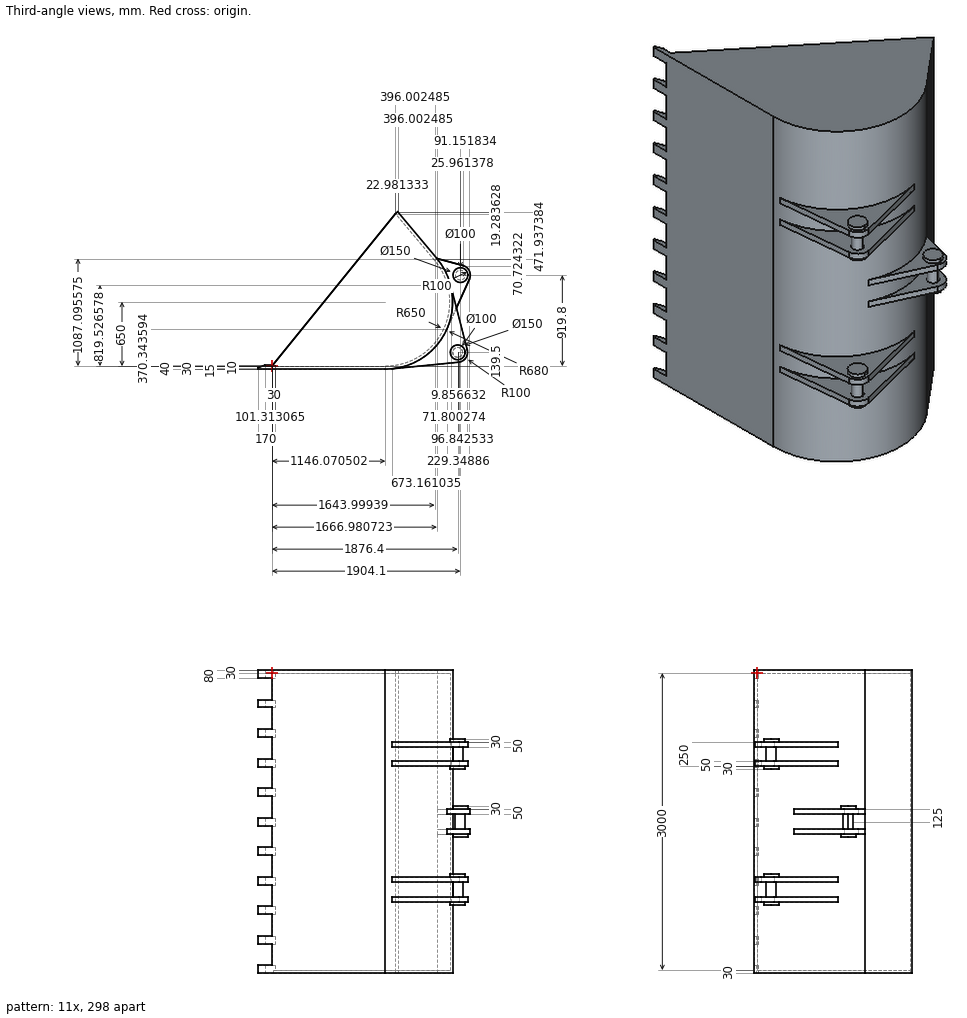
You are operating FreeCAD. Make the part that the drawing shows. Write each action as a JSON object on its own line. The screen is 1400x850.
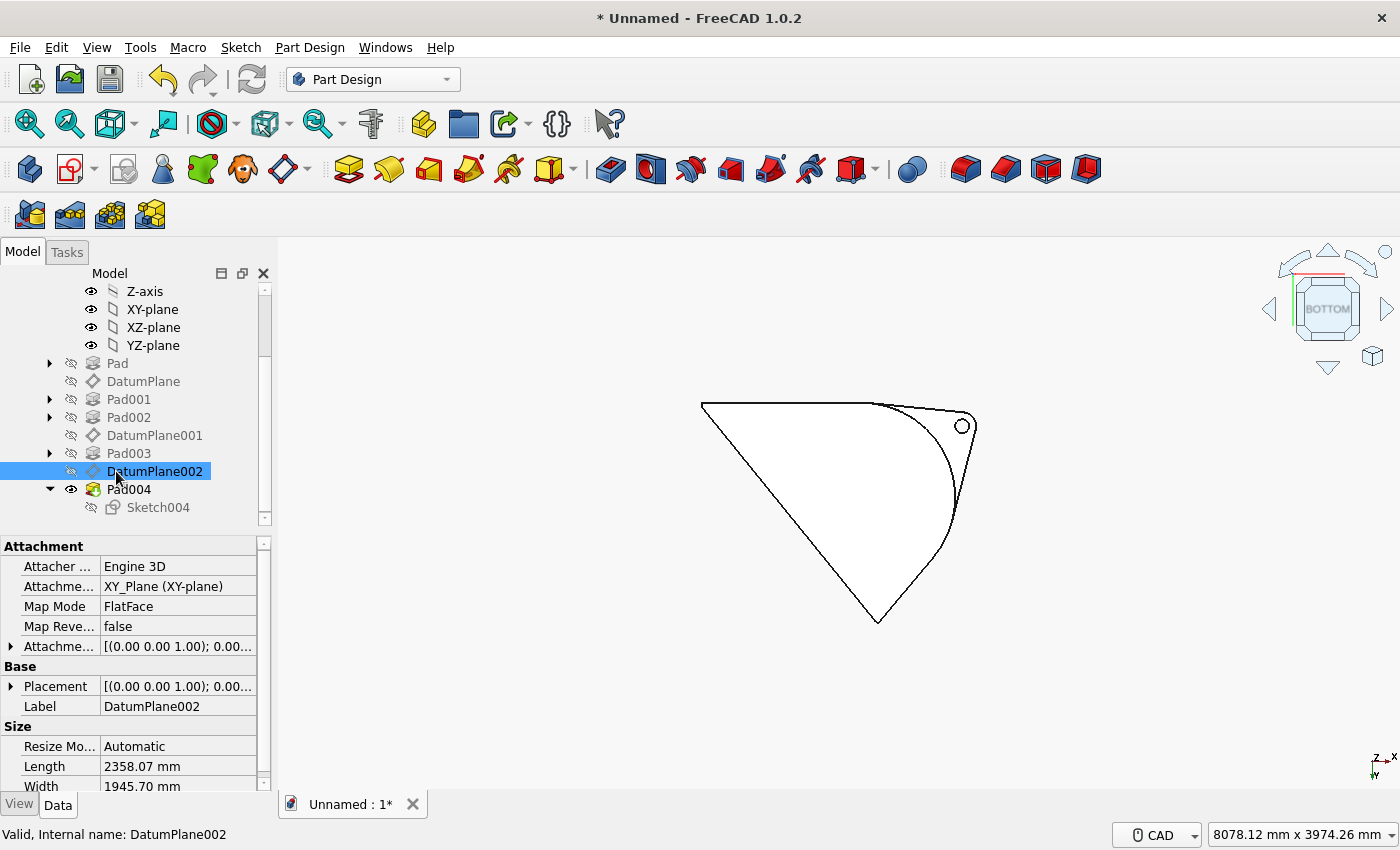
{"action": "left_click", "coordinate": [30, 124]}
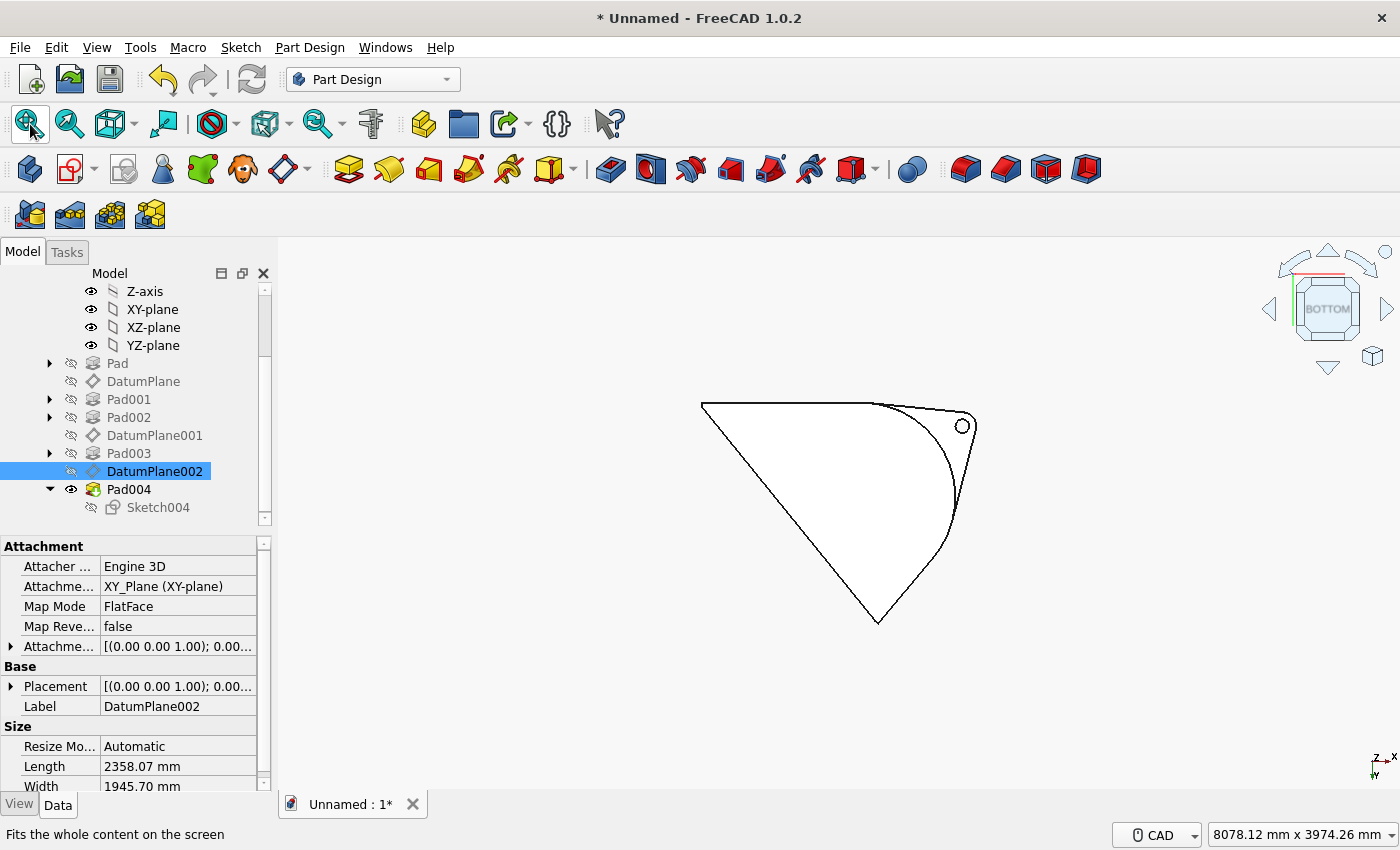
{"action": "scroll", "coordinate": [160, 395], "scroll_direction": "down", "scroll_amount": 3}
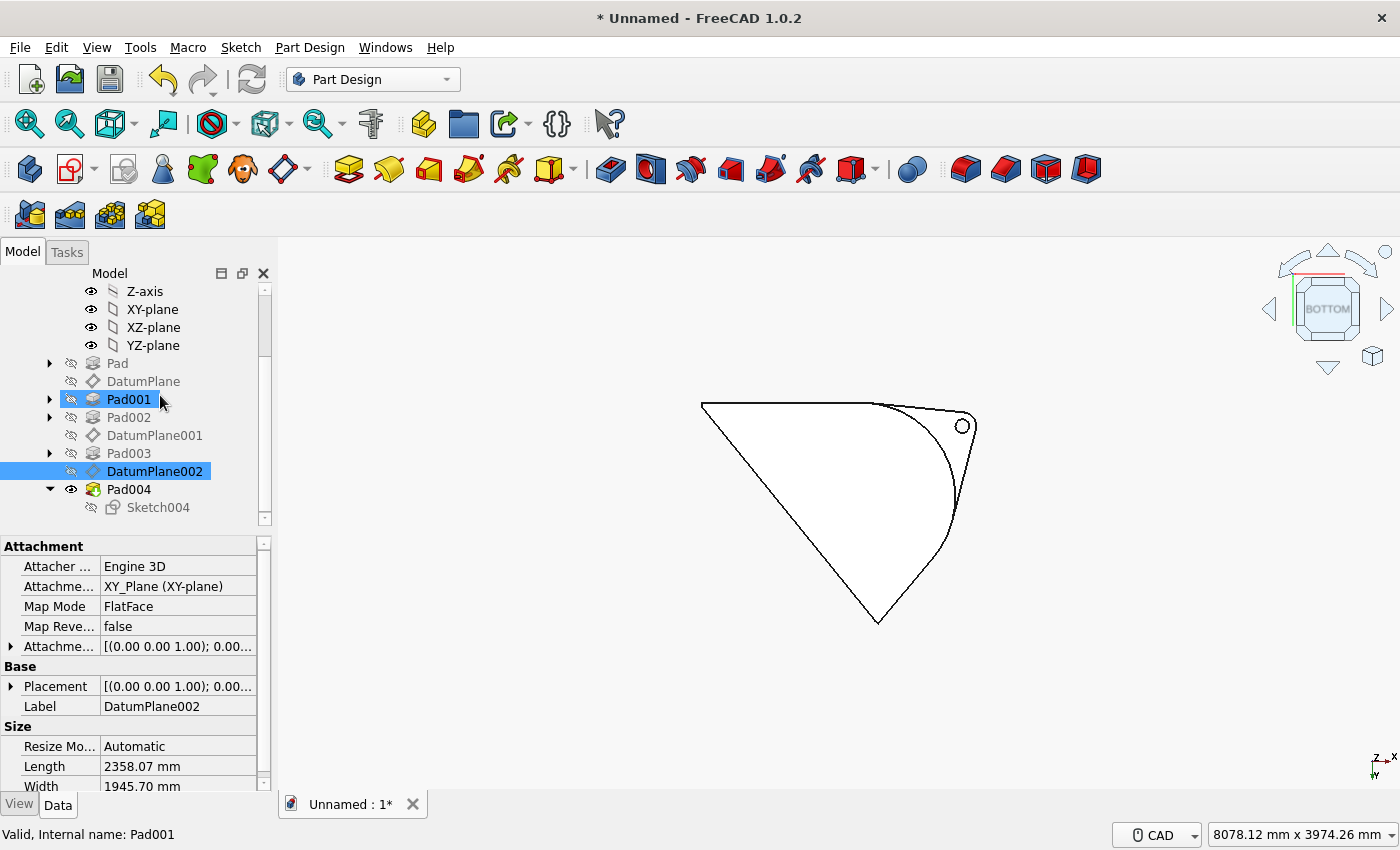
{"action": "scroll", "coordinate": [160, 395], "scroll_direction": "up", "scroll_amount": 15}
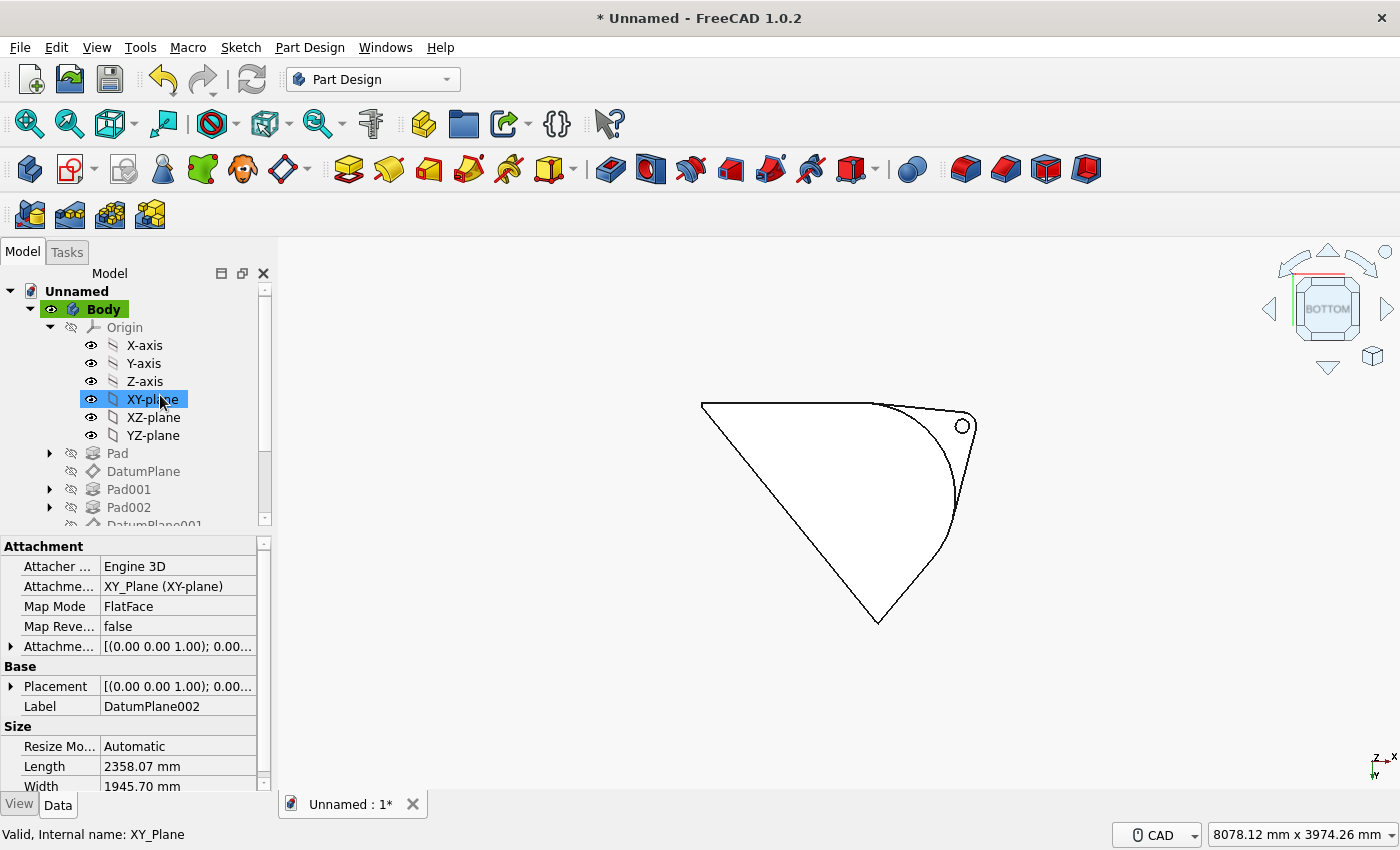
{"action": "left_click", "coordinate": [136, 399]}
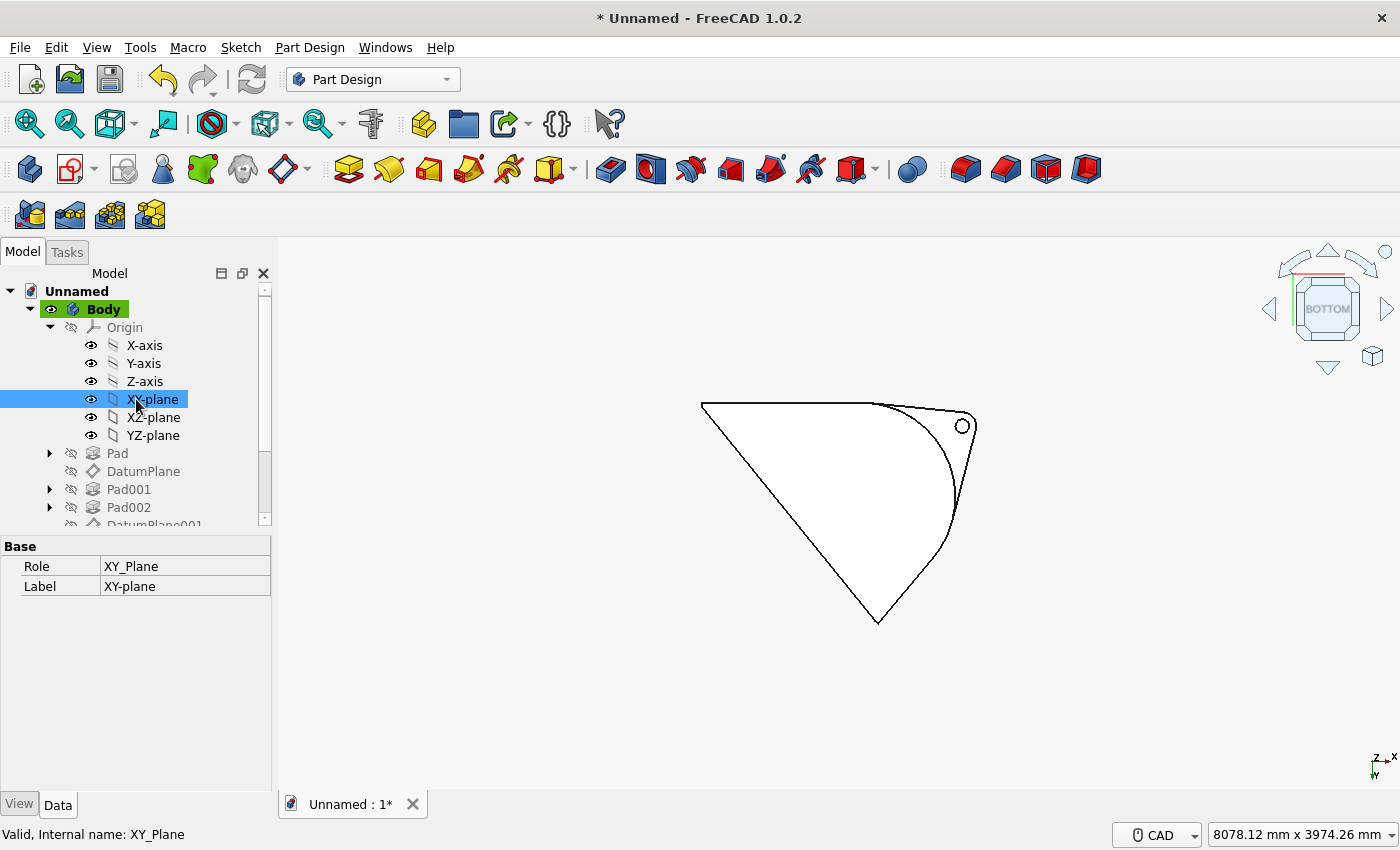
{"action": "left_click", "coordinate": [284, 170]}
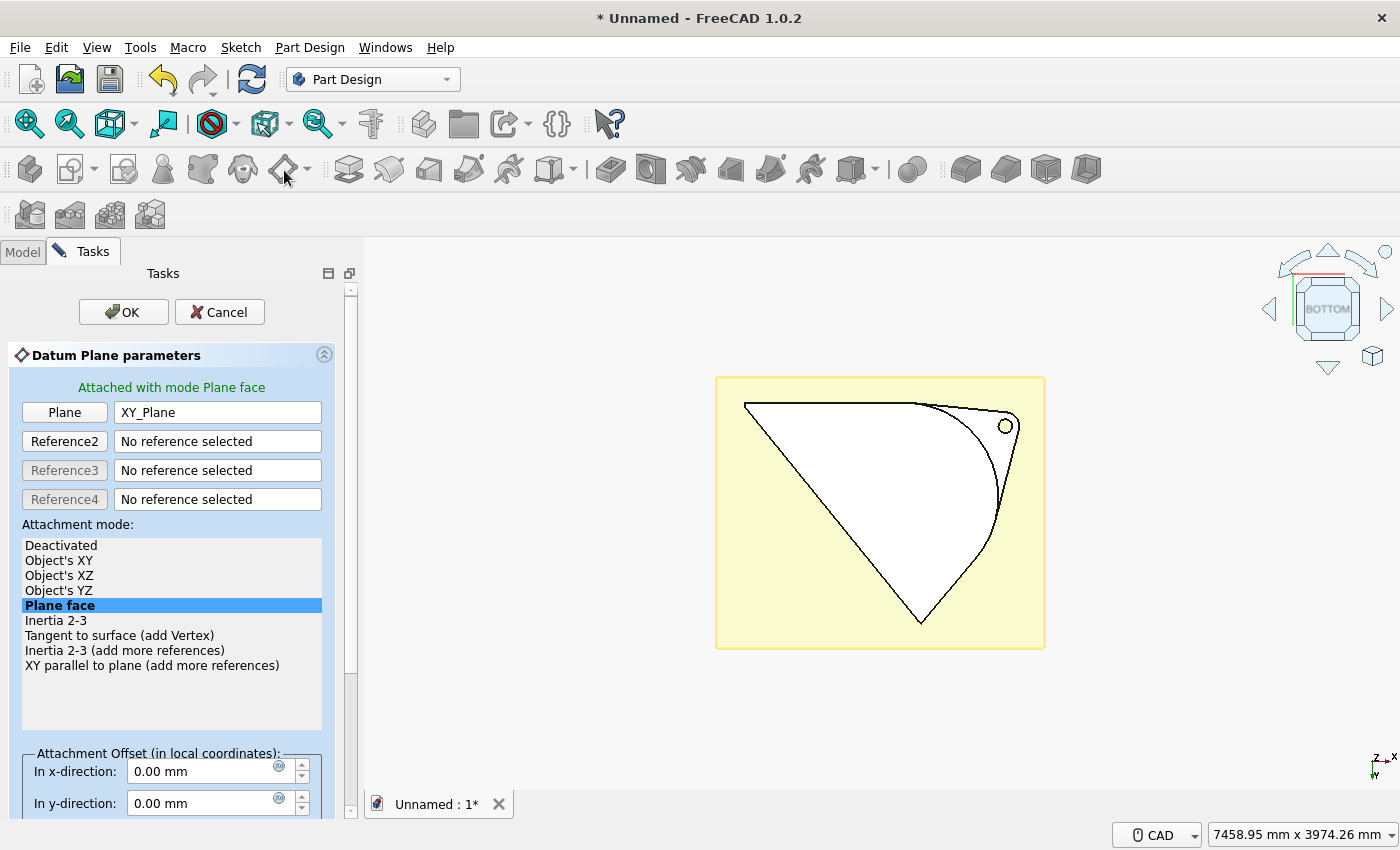
{"action": "scroll", "coordinate": [351, 550], "scroll_direction": "down", "scroll_amount": 2}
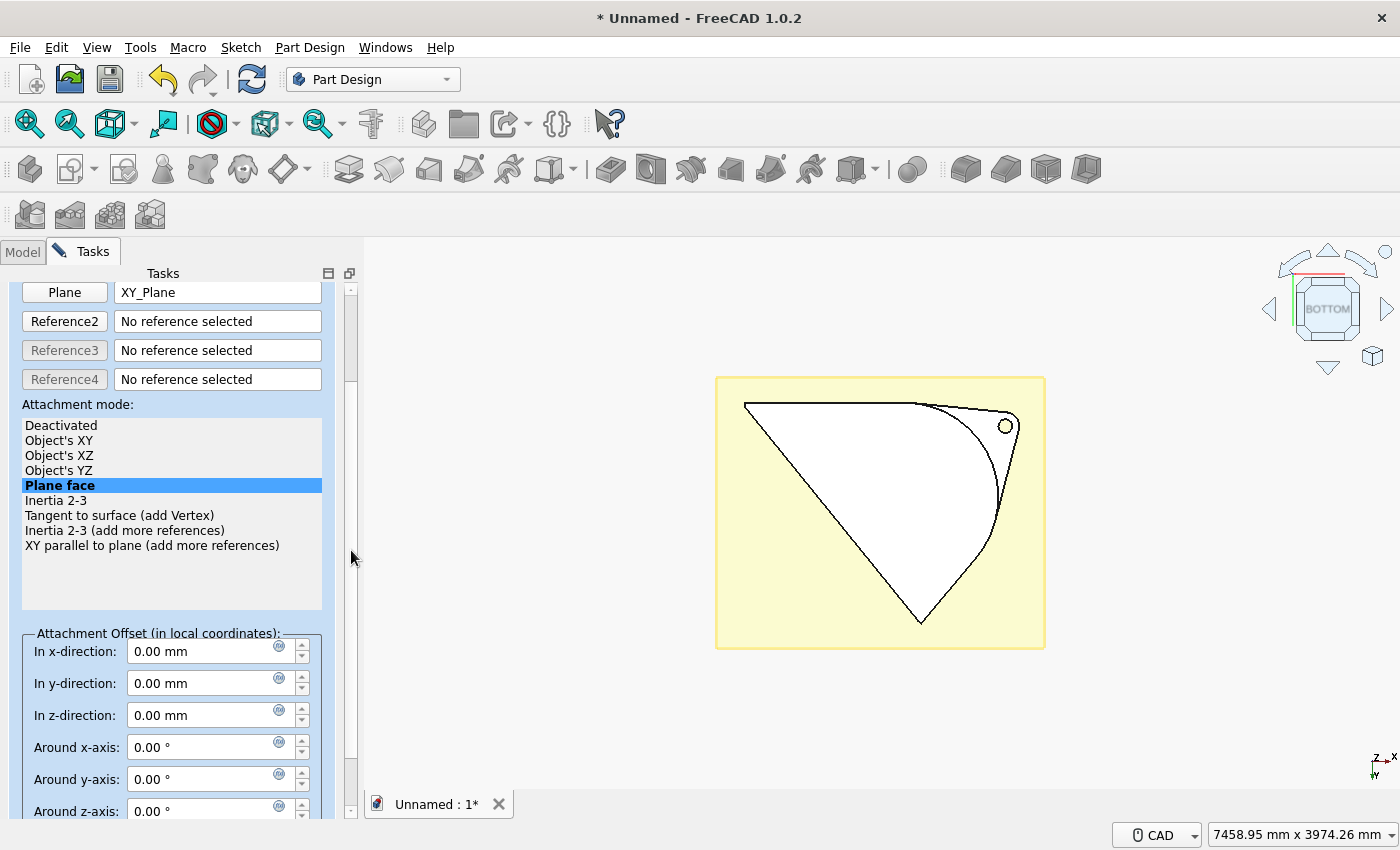
{"action": "triple_click", "coordinate": [210, 715]}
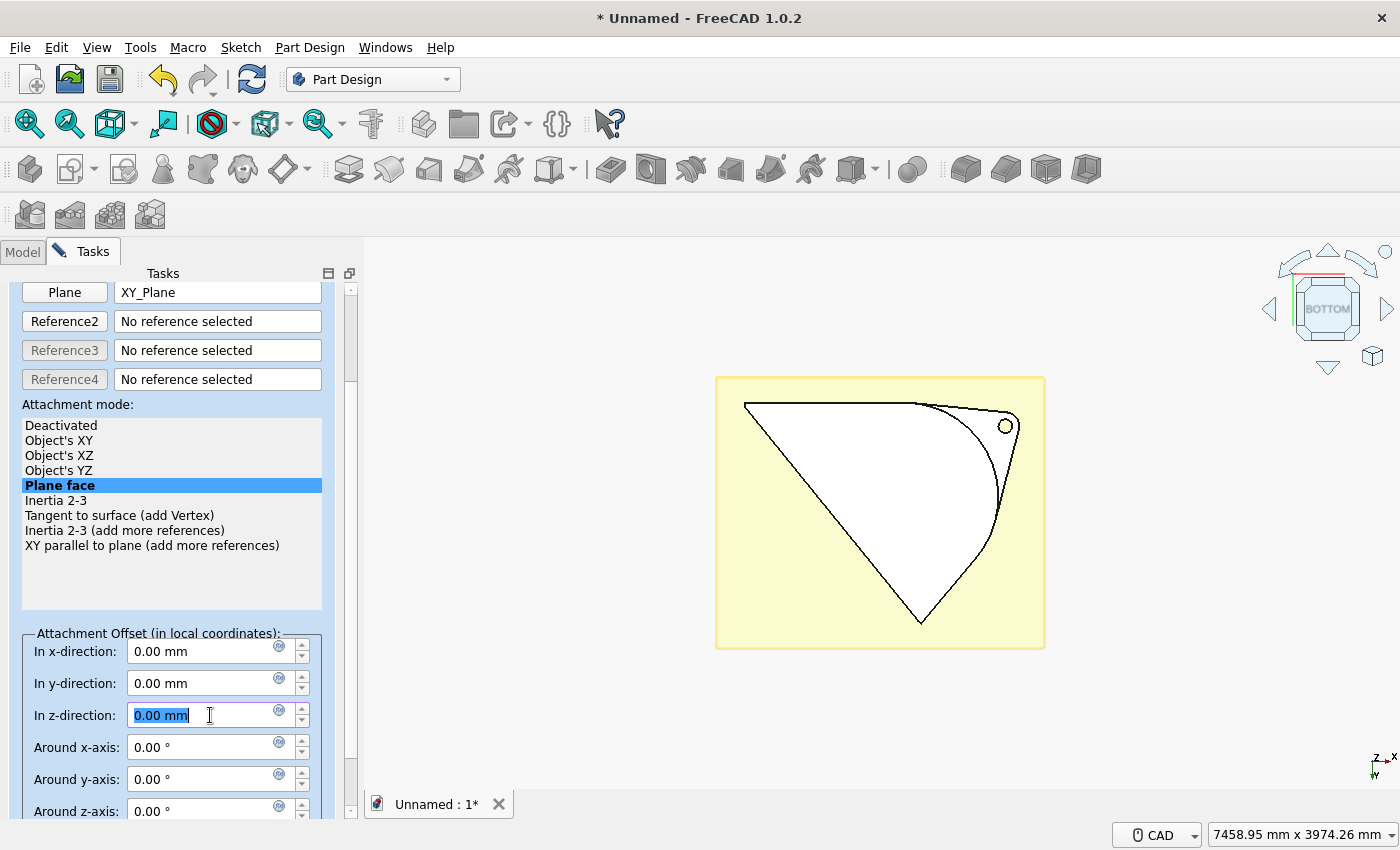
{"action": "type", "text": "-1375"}
{"action": "key", "text": "Tab"}